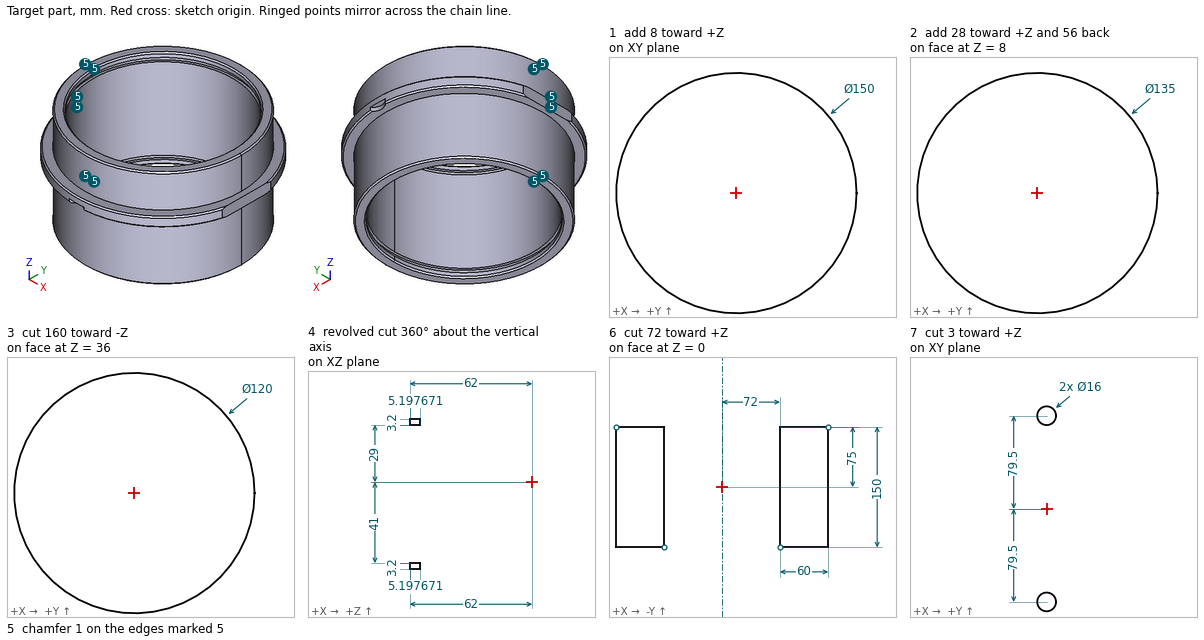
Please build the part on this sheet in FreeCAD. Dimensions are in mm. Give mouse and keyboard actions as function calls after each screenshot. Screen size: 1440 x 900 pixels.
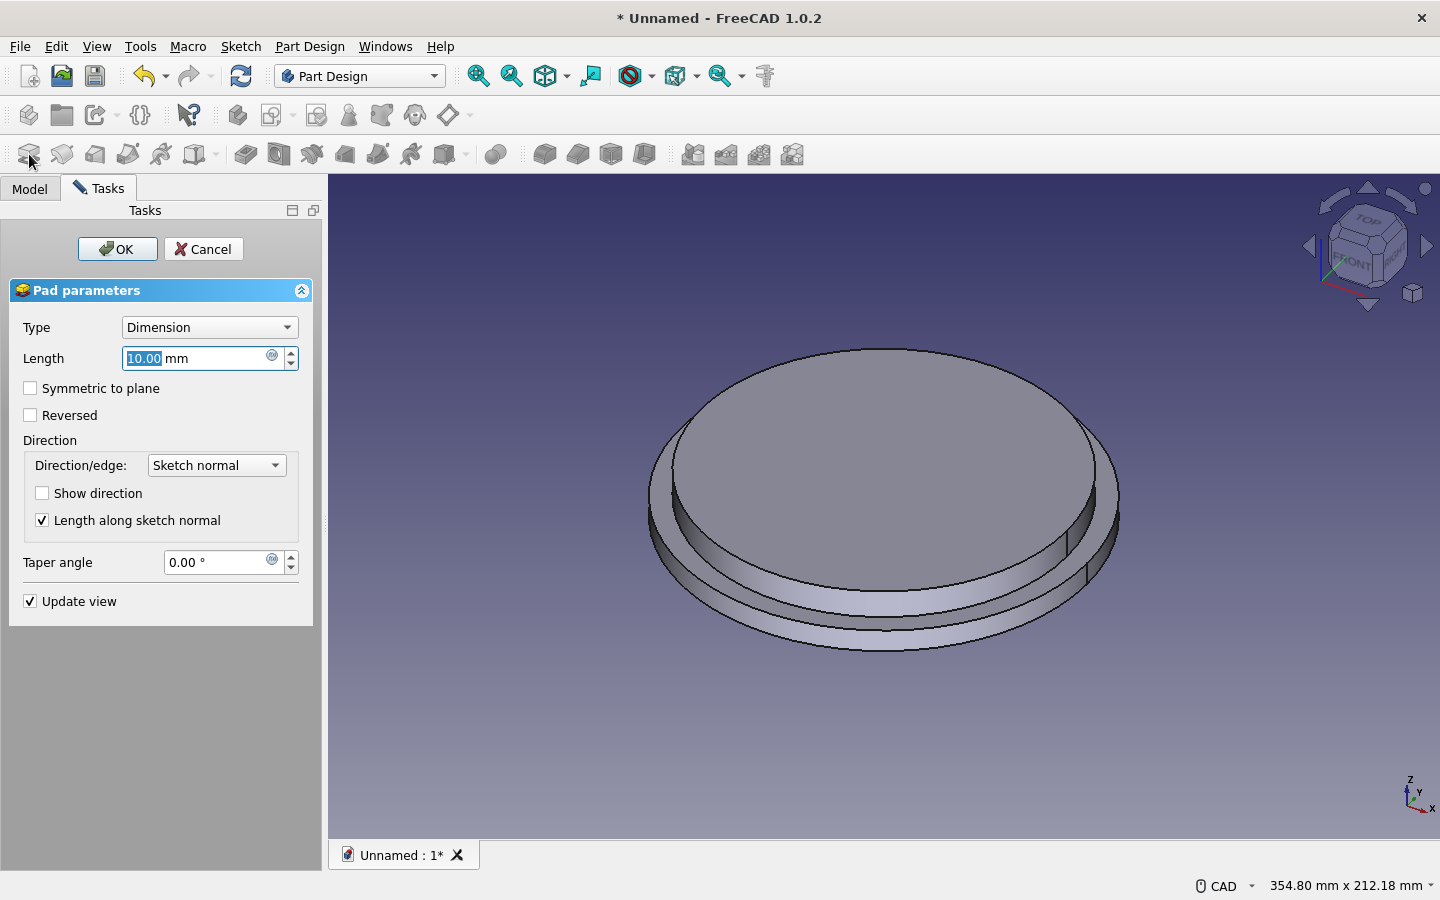
click(210, 328)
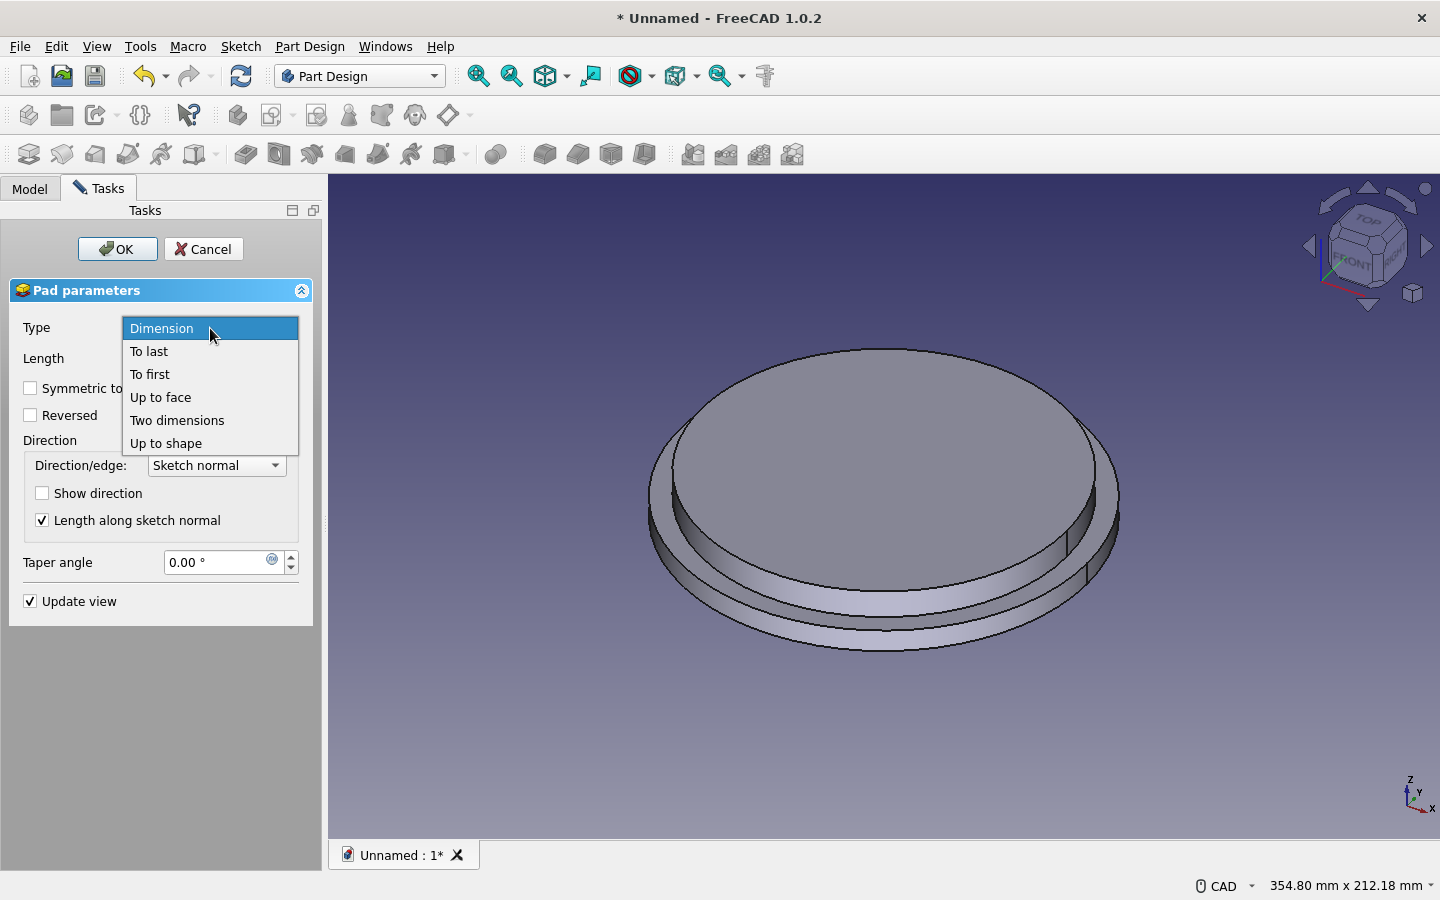
click(208, 420)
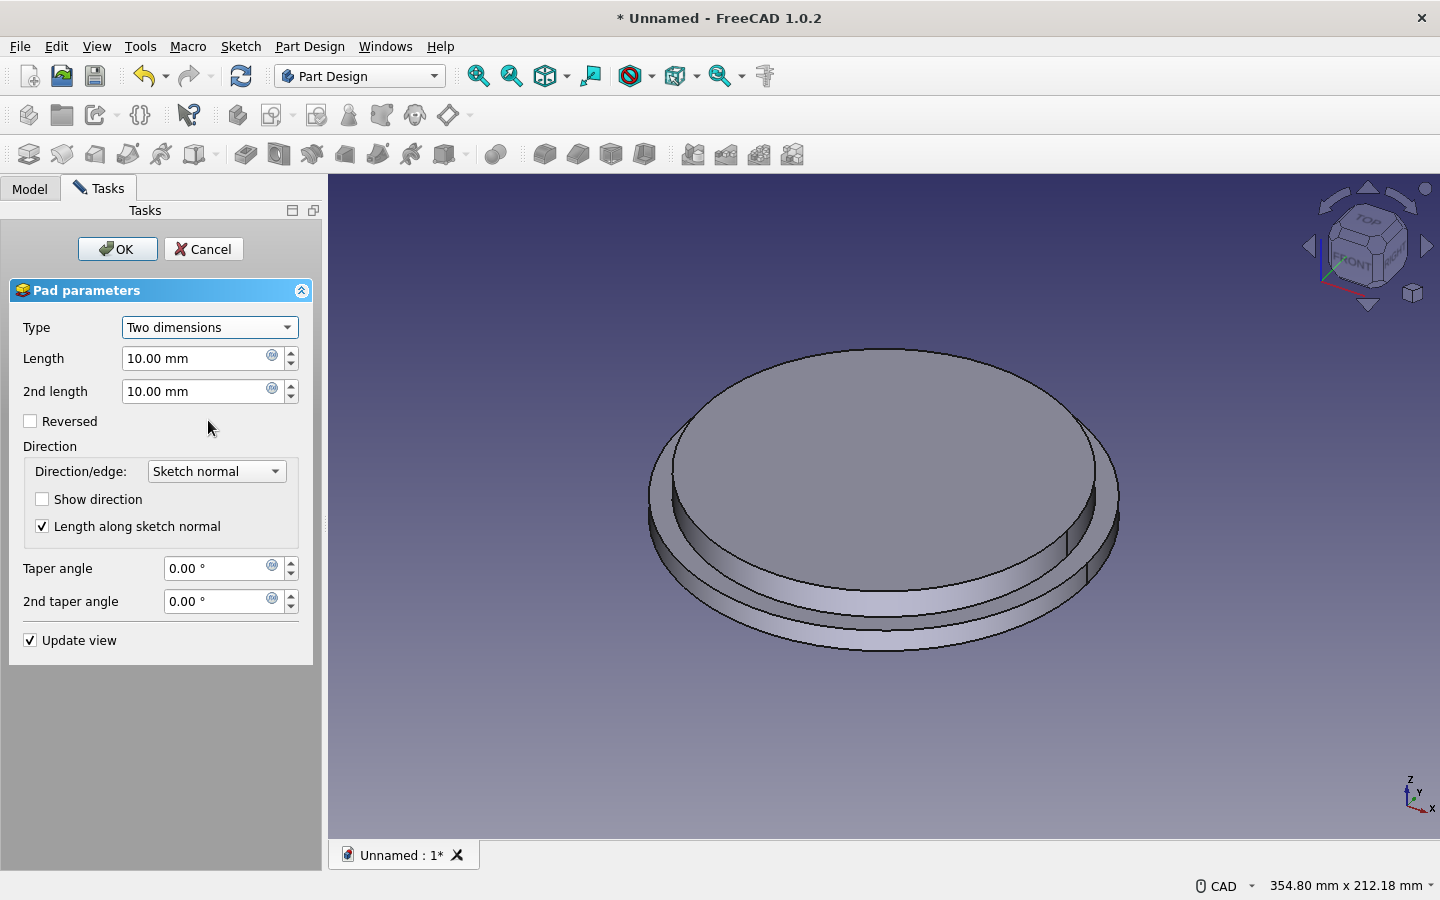
triple_click(204, 358)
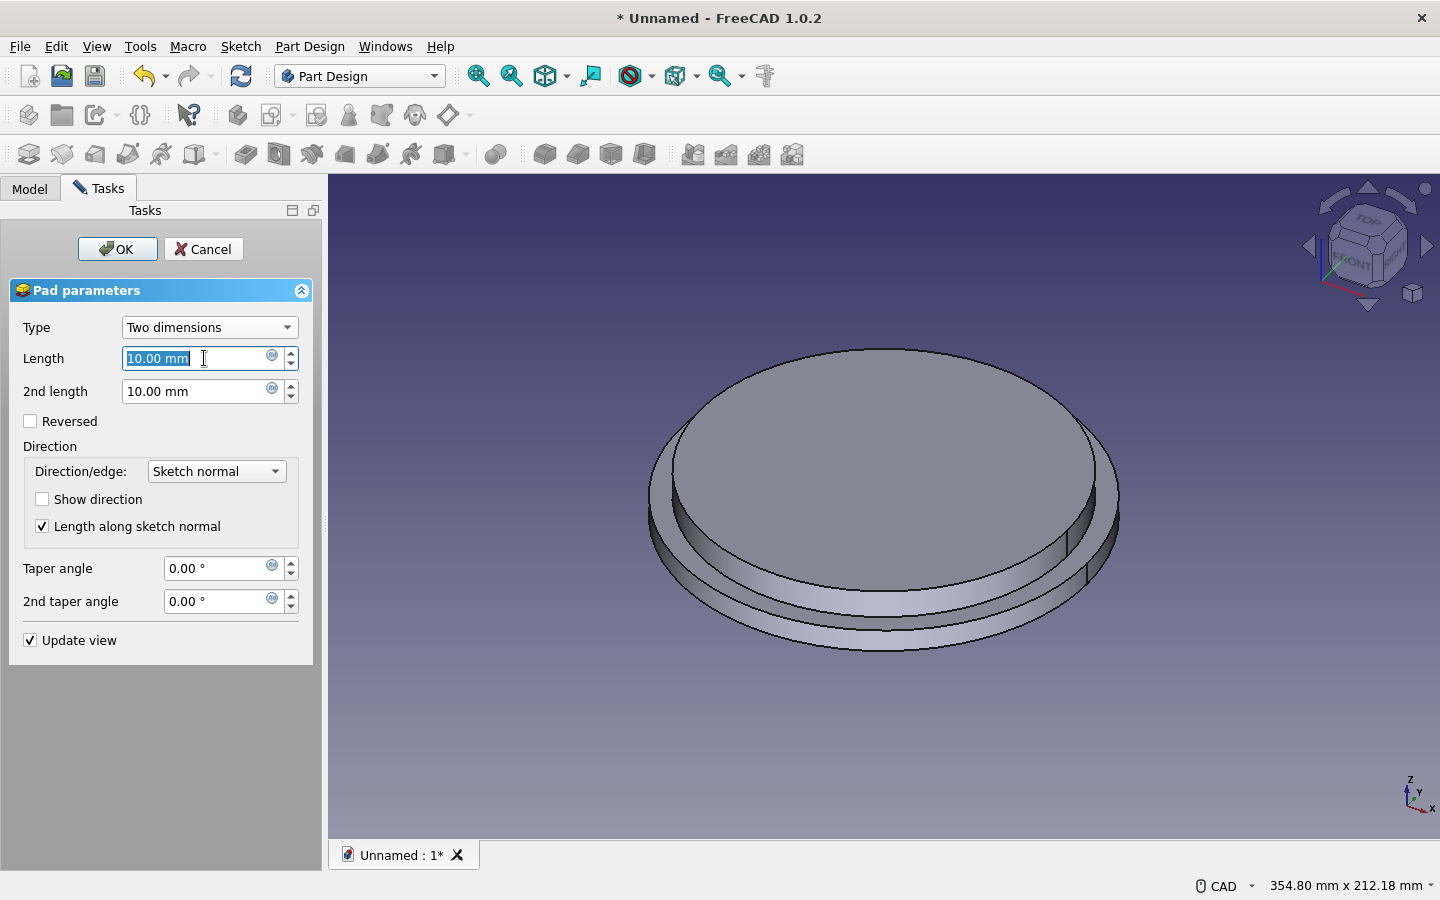
text(28)
key(Tab)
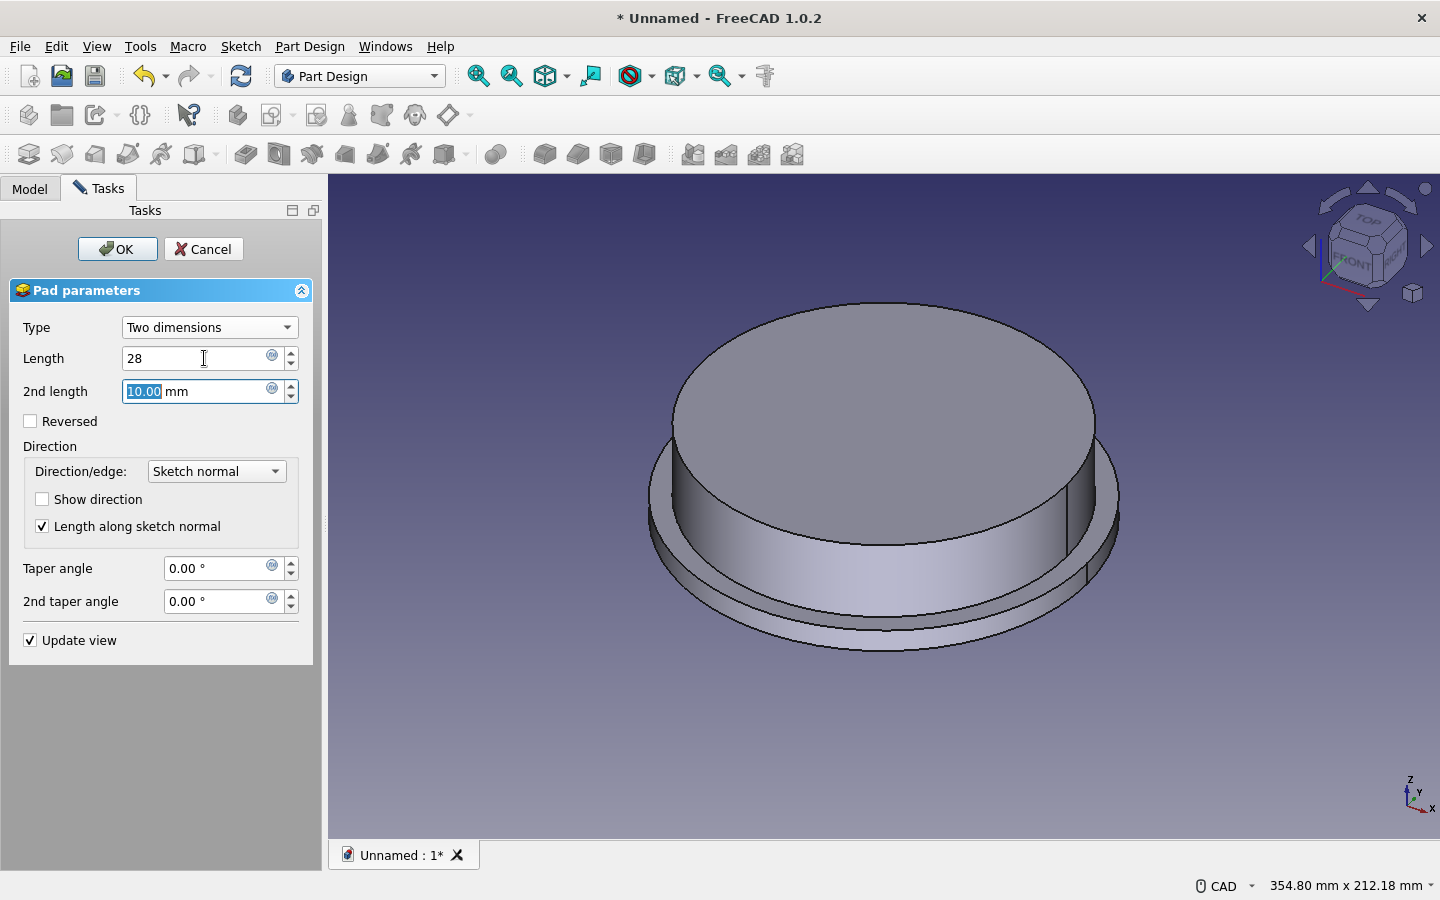
text(56)
key(Tab)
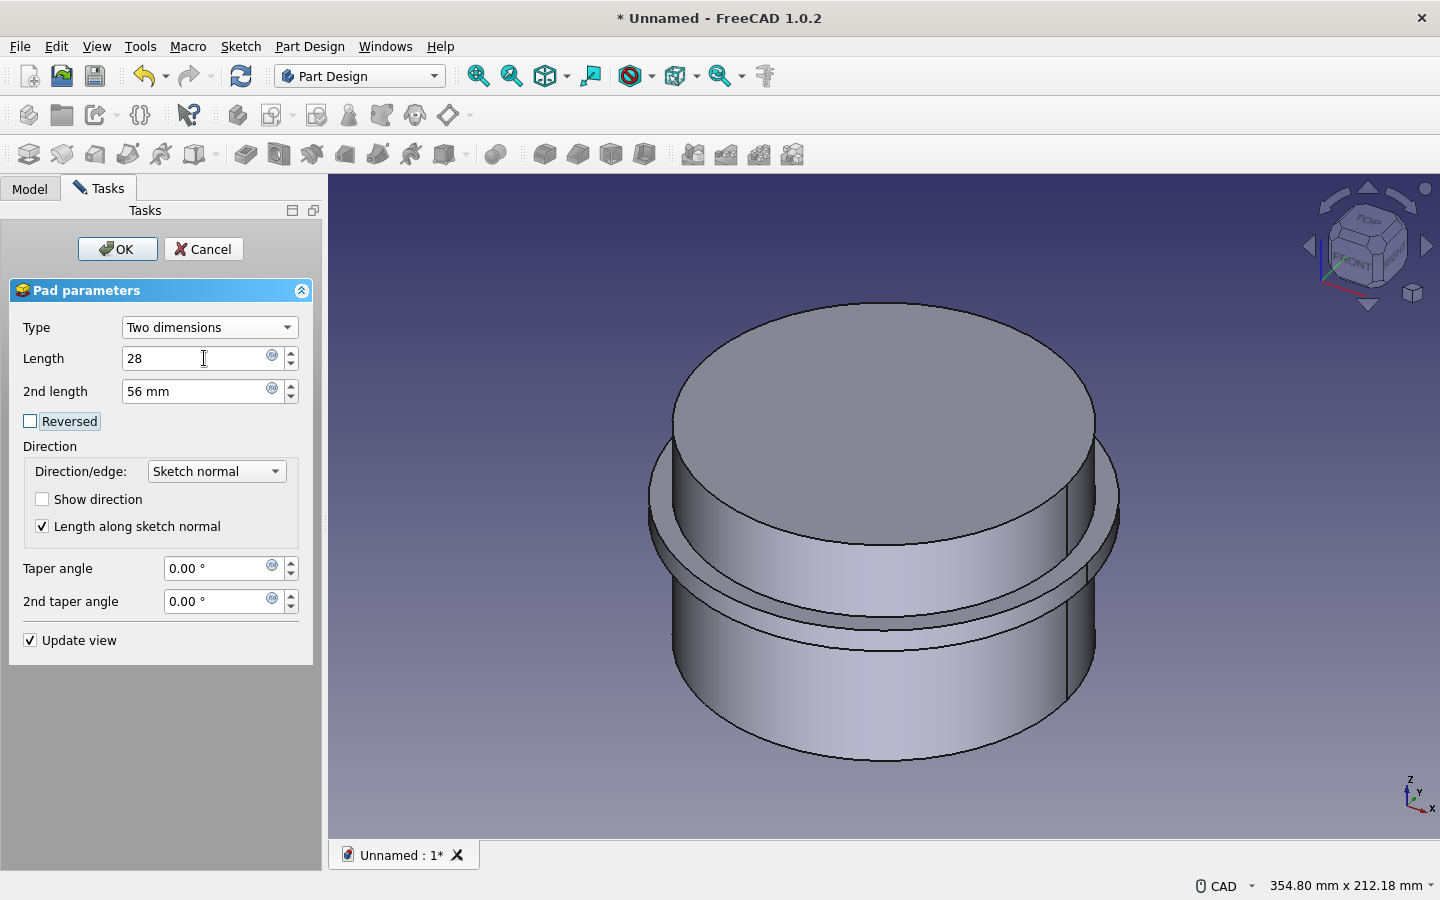
click(118, 249)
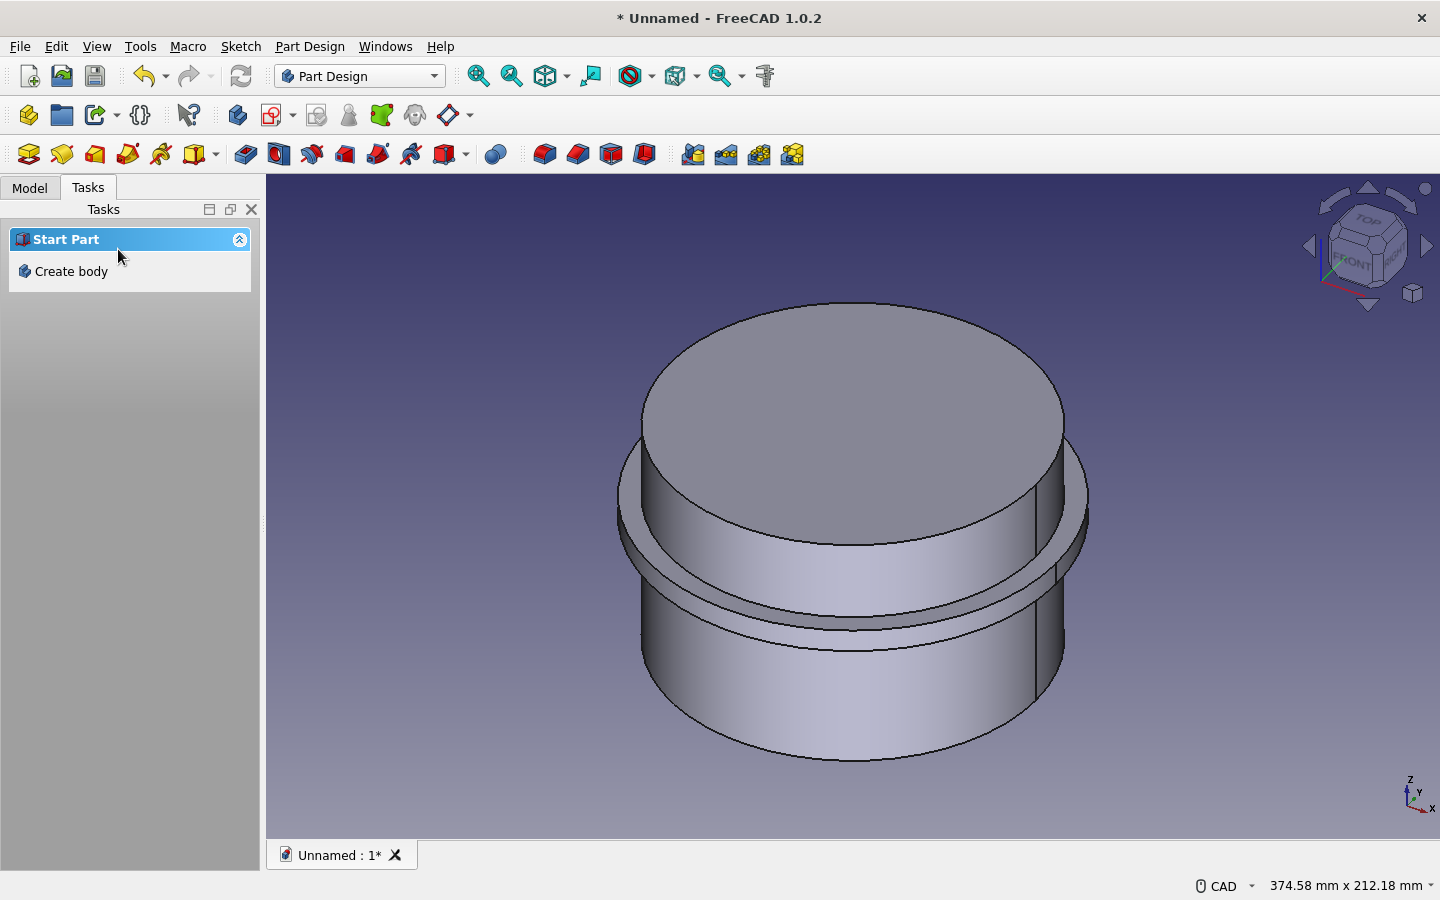
click(853, 423)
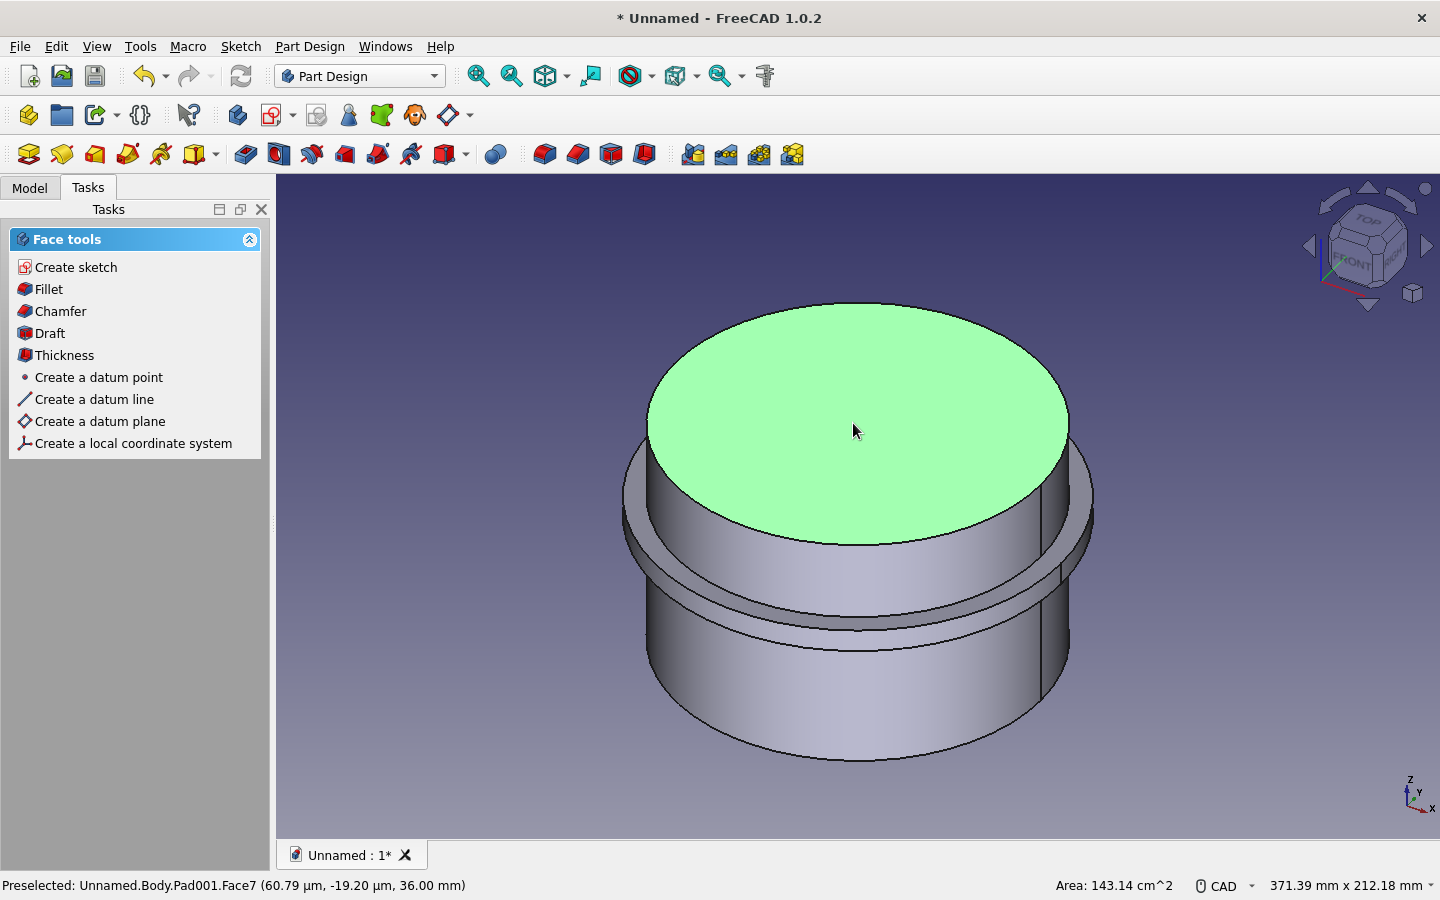
click(270, 116)